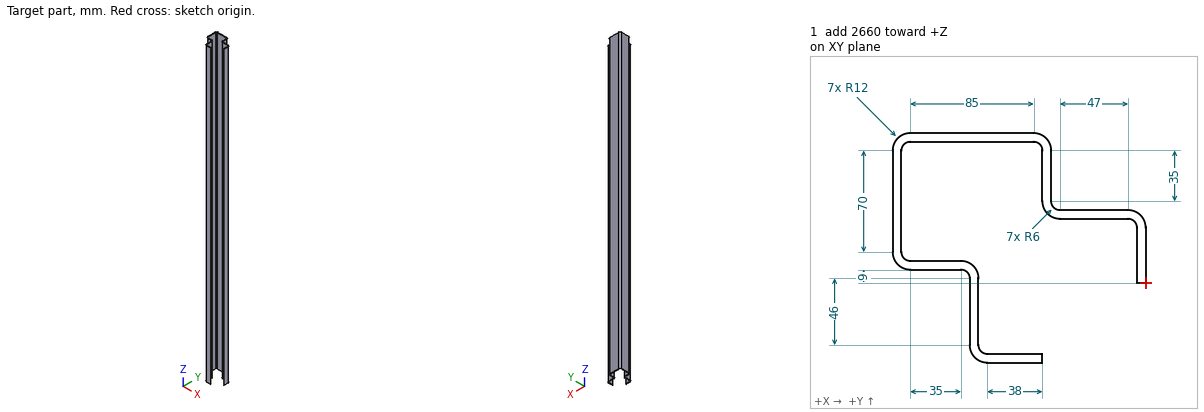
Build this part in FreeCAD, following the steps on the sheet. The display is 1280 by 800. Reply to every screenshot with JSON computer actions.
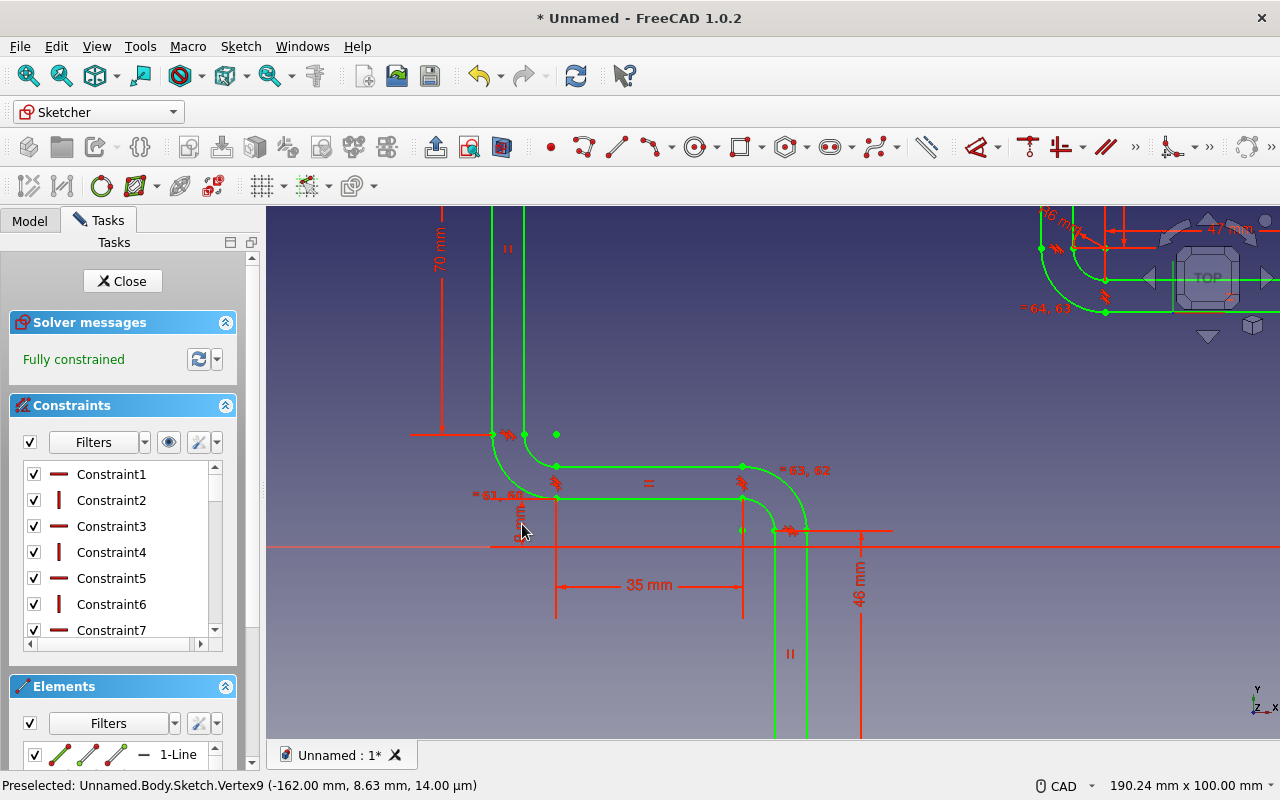
{"action": "left_click", "coordinate": [123, 281]}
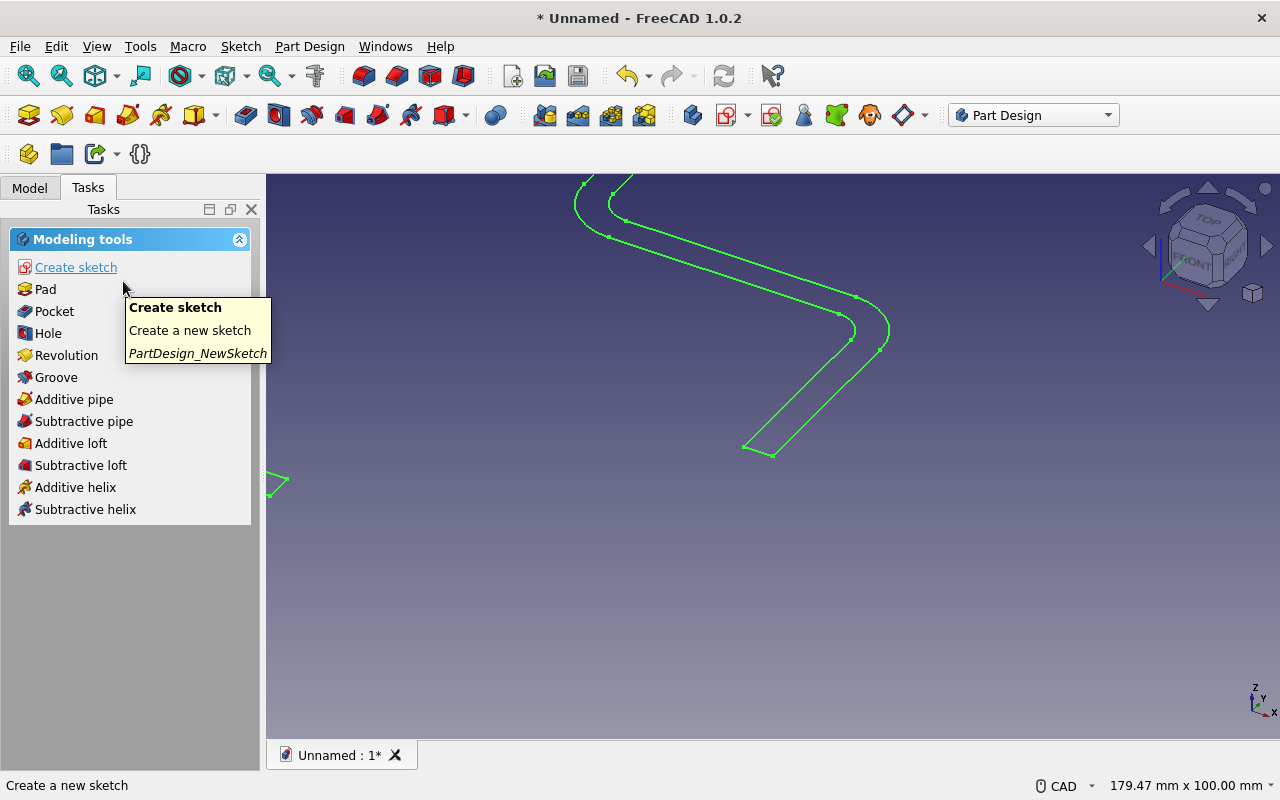
{"action": "left_click", "coordinate": [29, 116]}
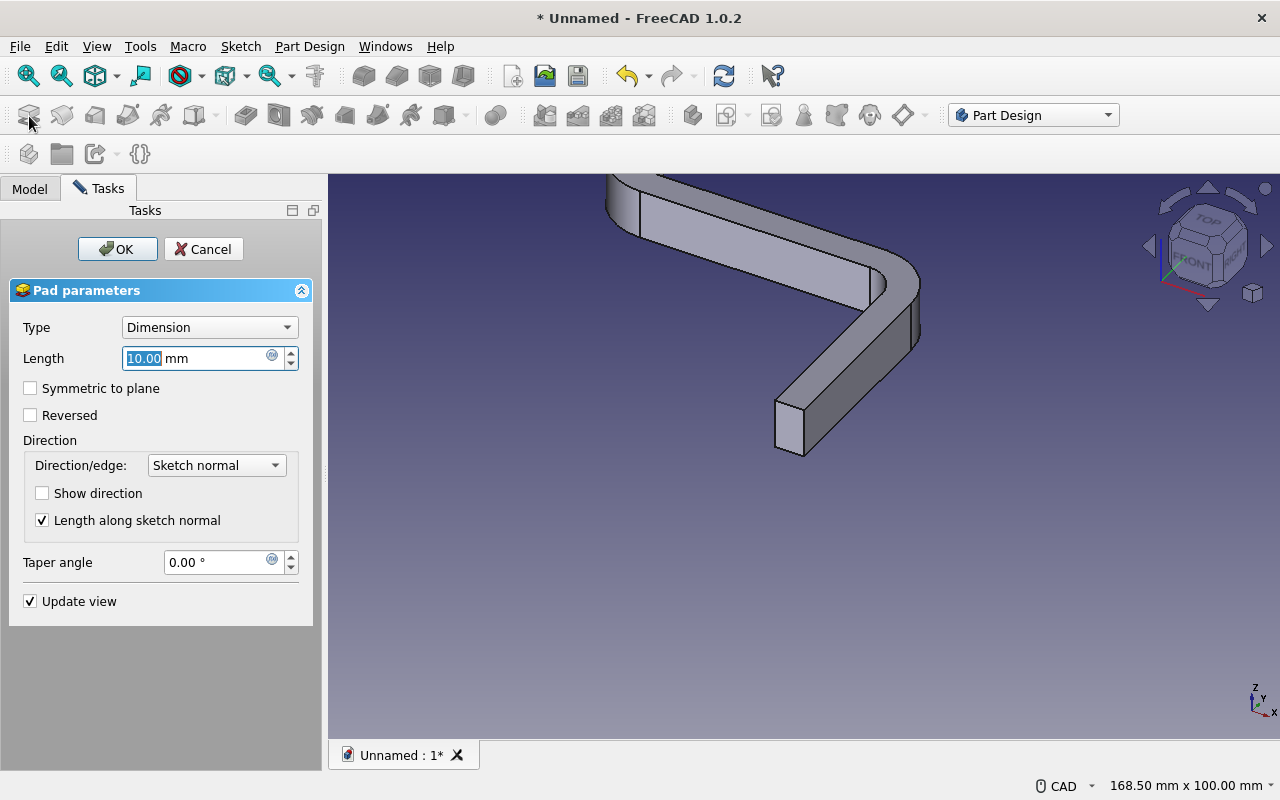
{"action": "type", "text": "2660"}
{"action": "key", "text": "Tab"}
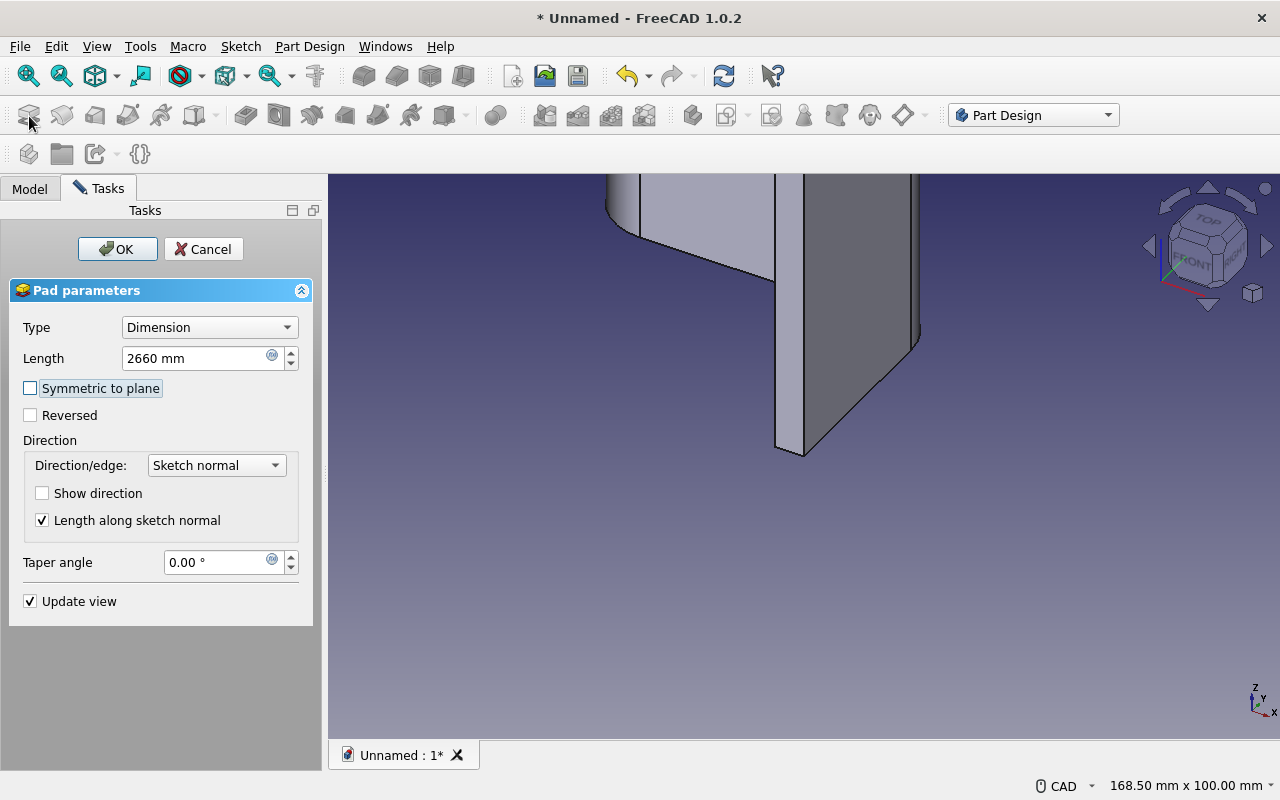
{"action": "left_click", "coordinate": [118, 249]}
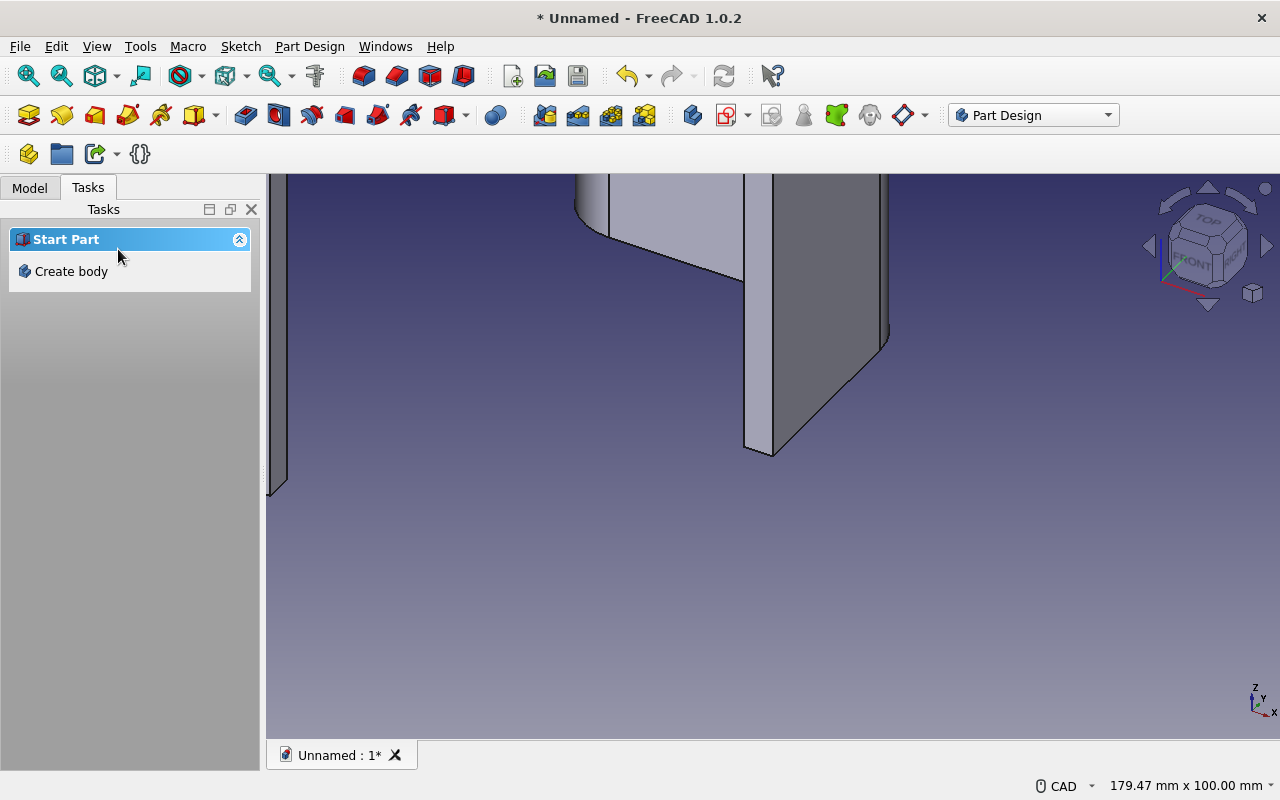
{"action": "key", "text": "0"}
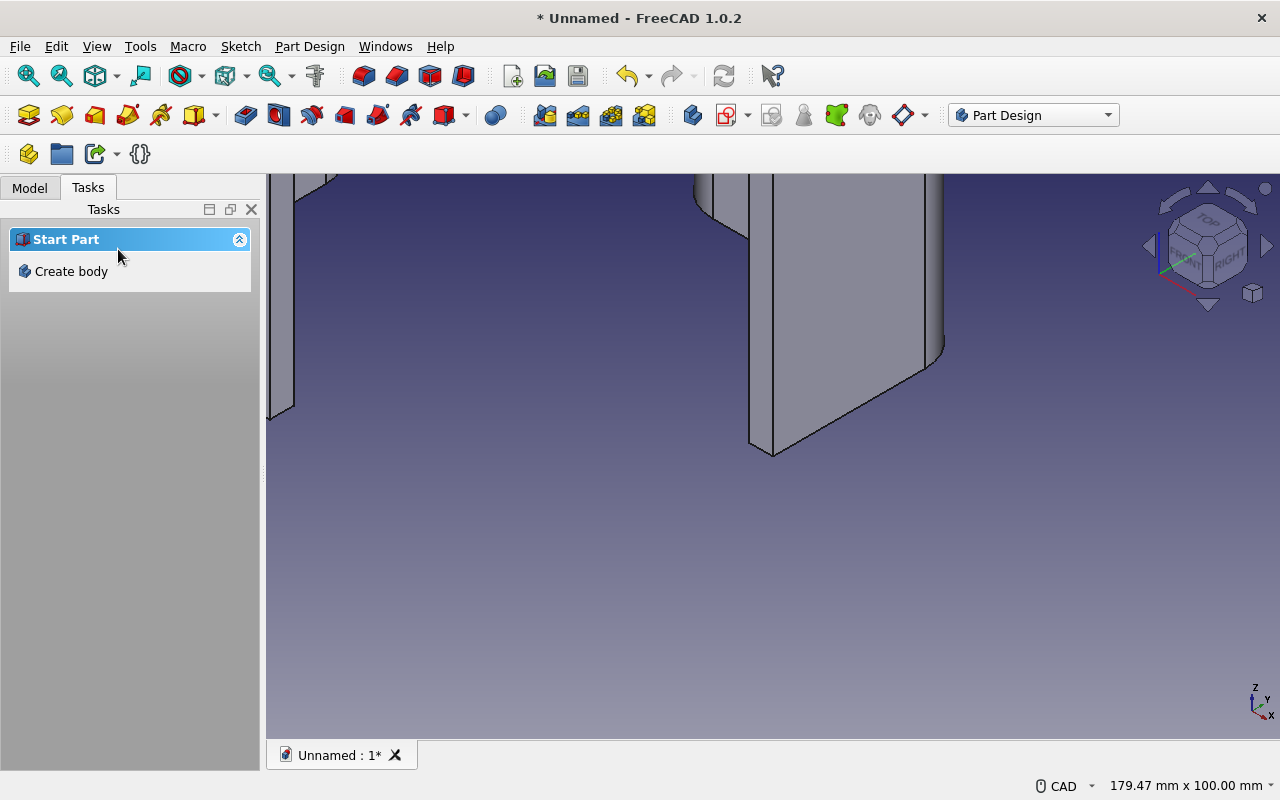
{"action": "key", "text": "v f"}